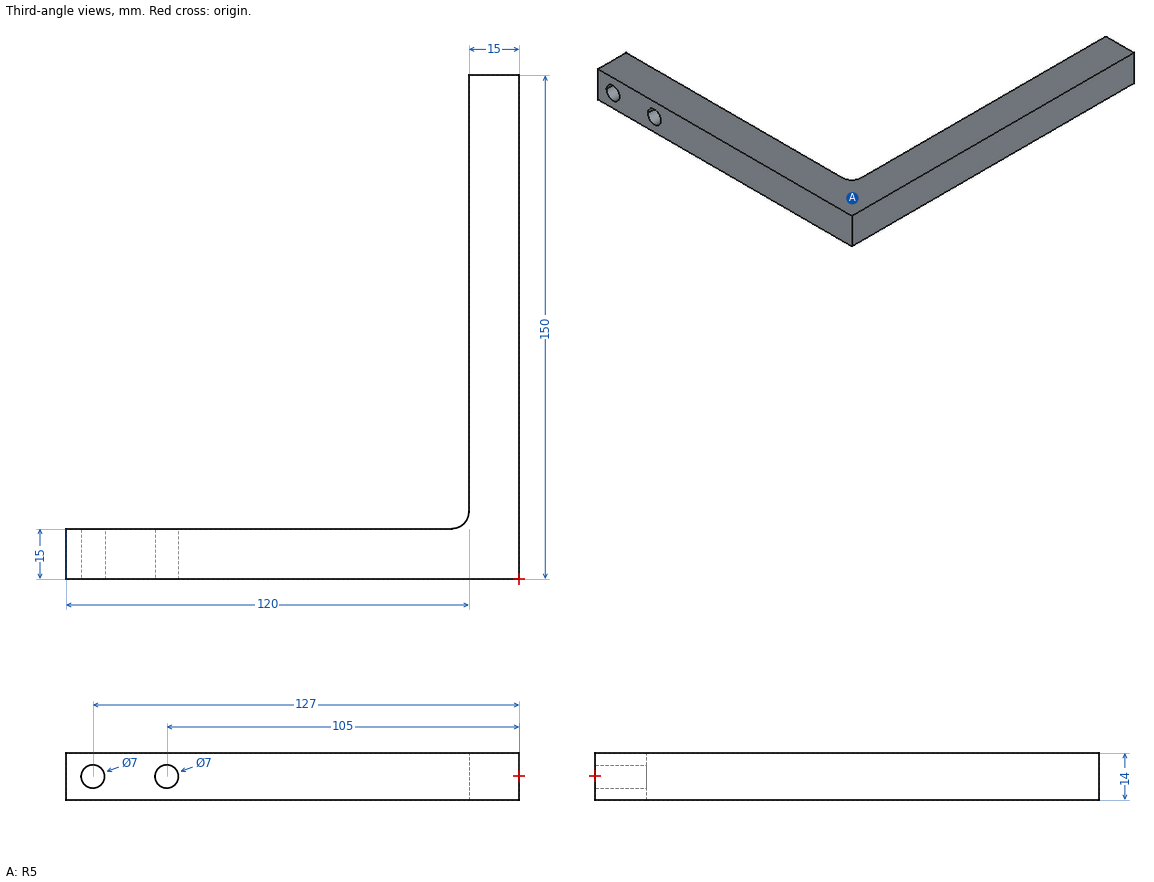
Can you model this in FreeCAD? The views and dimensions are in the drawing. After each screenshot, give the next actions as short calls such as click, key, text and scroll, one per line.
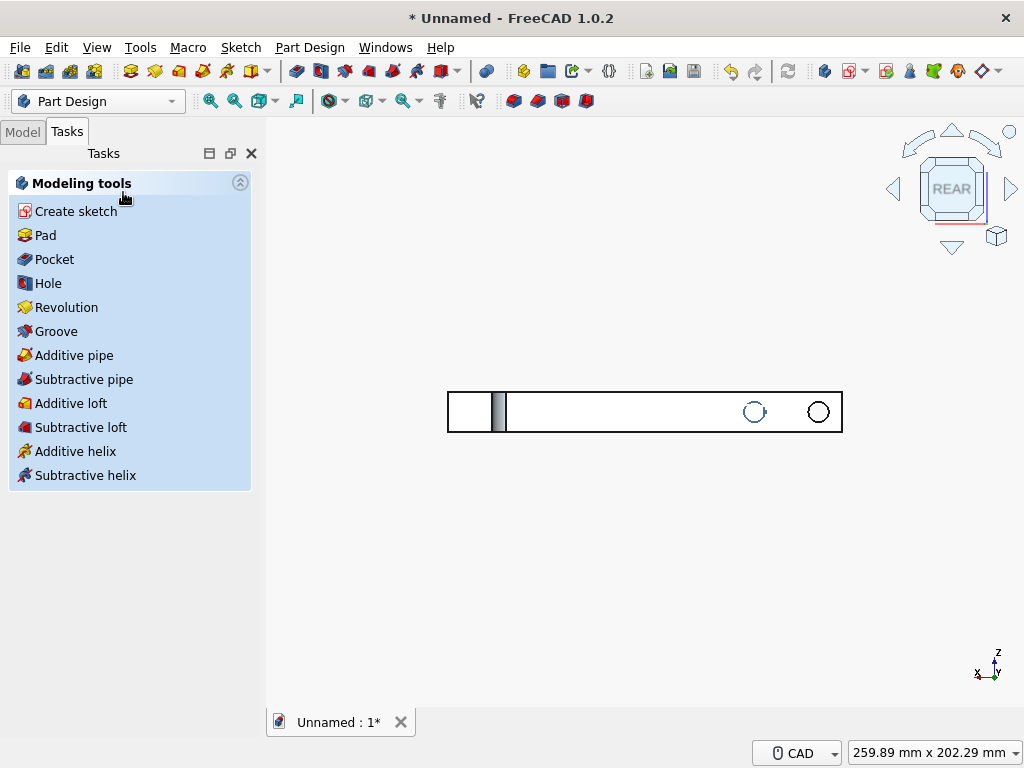
click(298, 72)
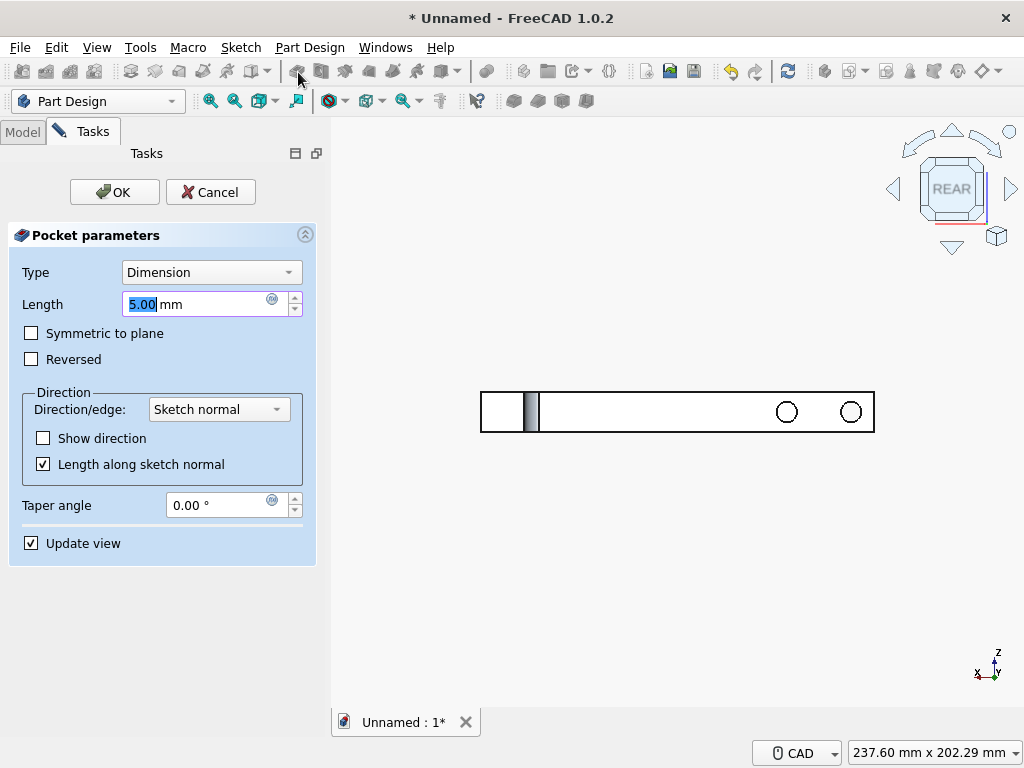
click(212, 272)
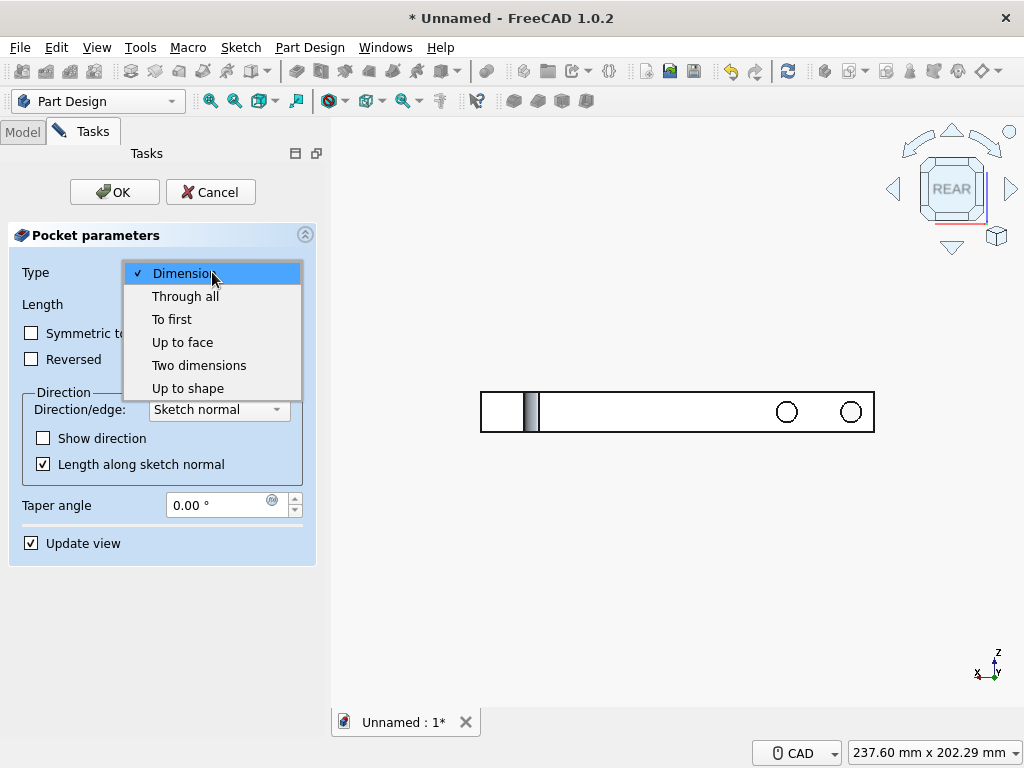
click(212, 320)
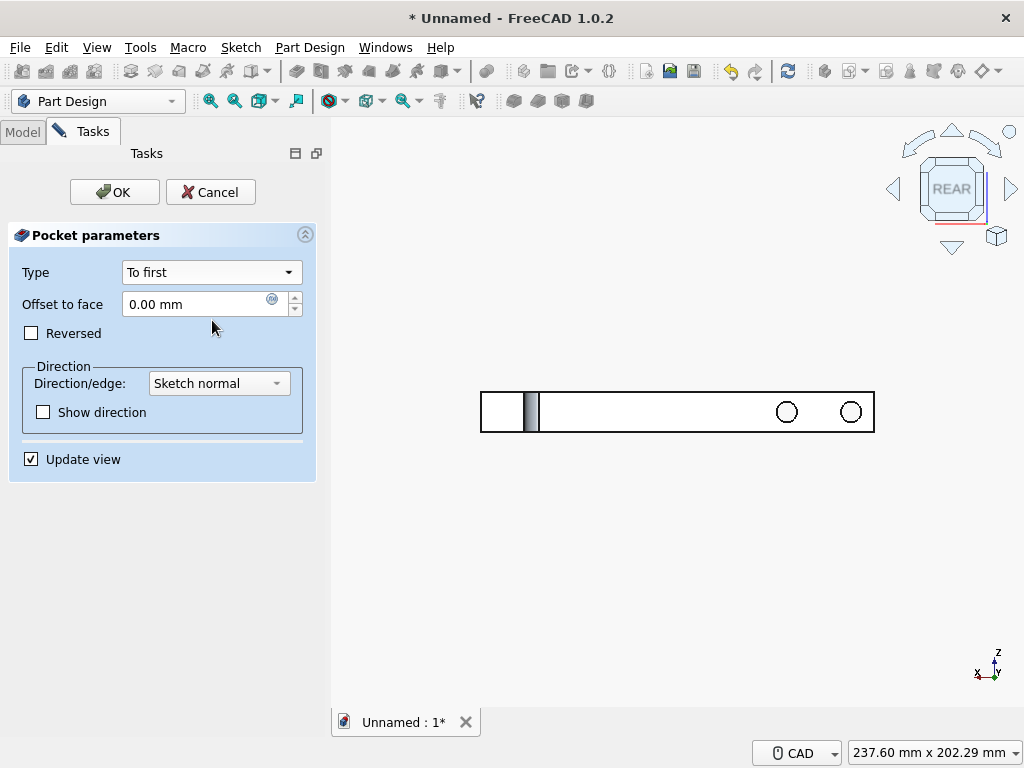
click(115, 192)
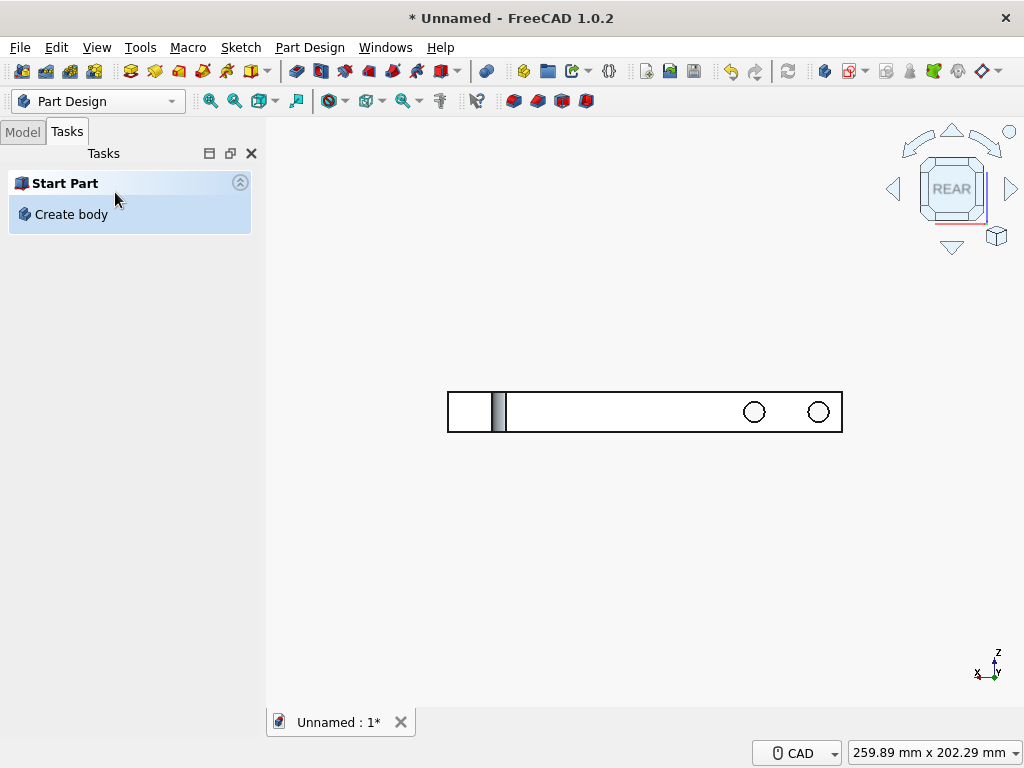
key(0)